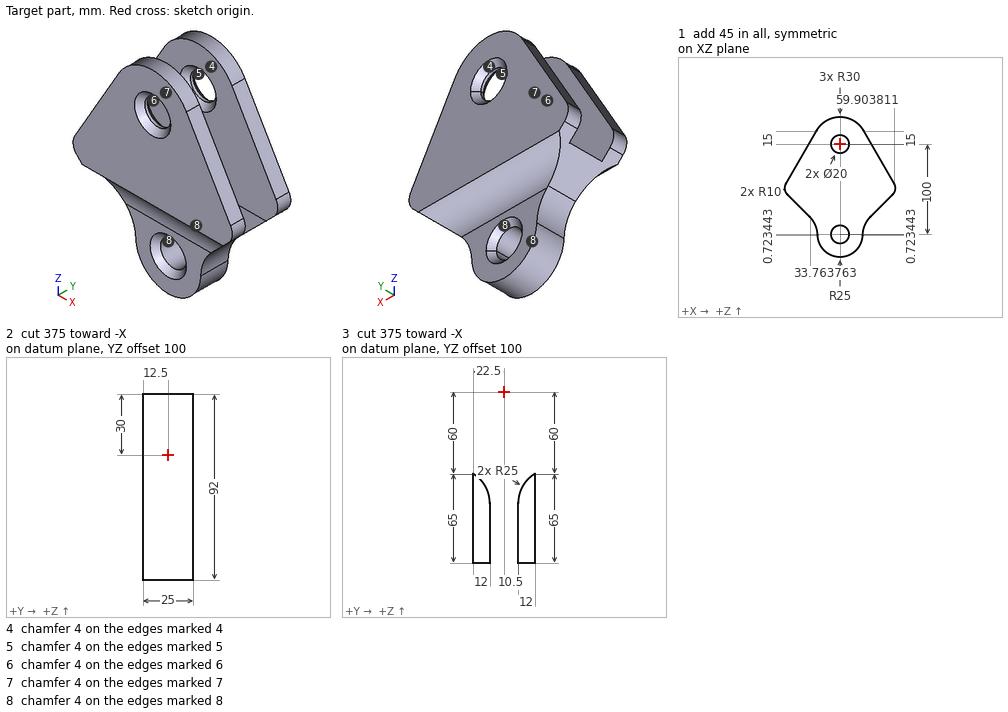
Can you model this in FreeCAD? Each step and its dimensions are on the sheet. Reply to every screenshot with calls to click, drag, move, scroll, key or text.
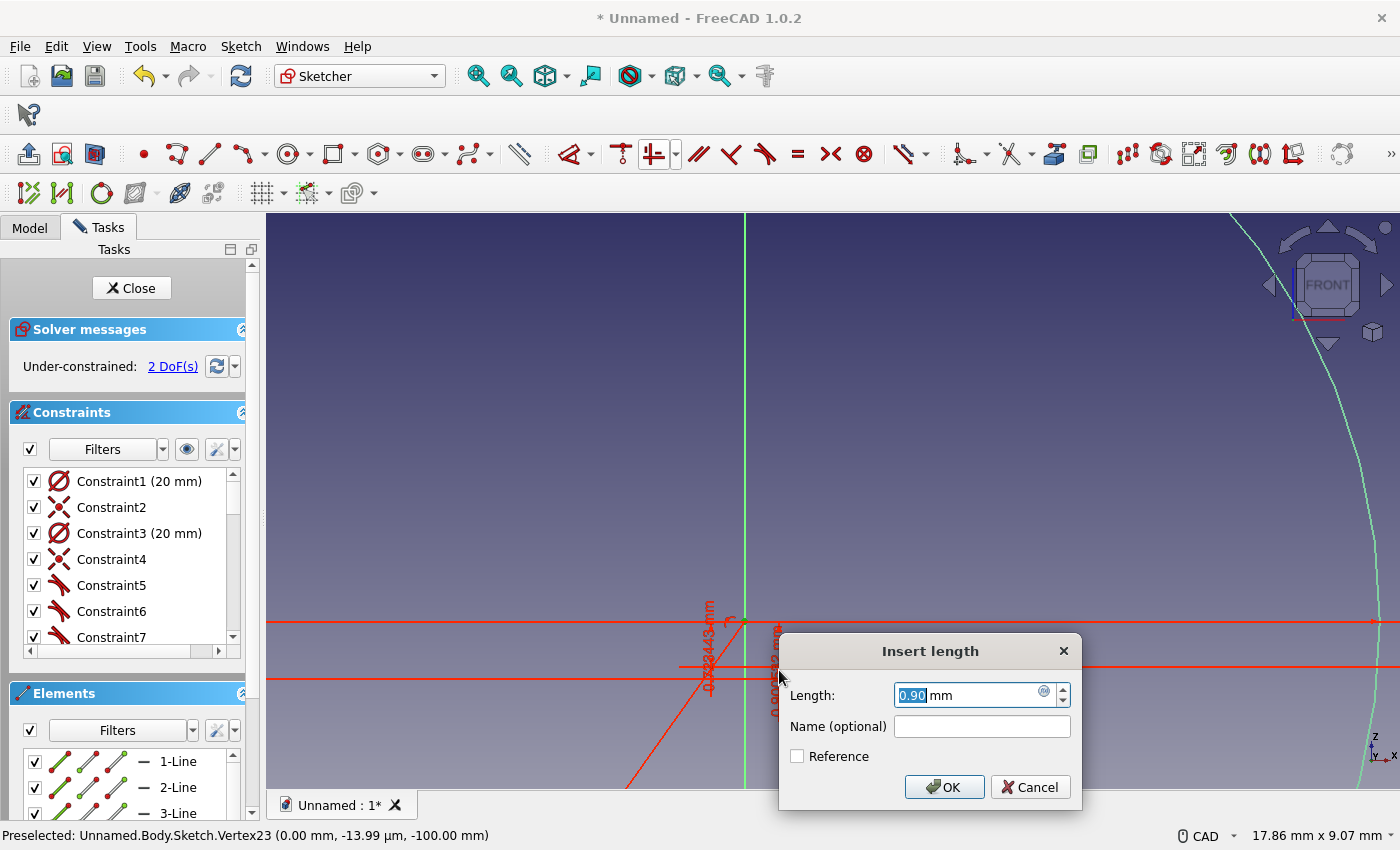
text(0.723443)
key(Return)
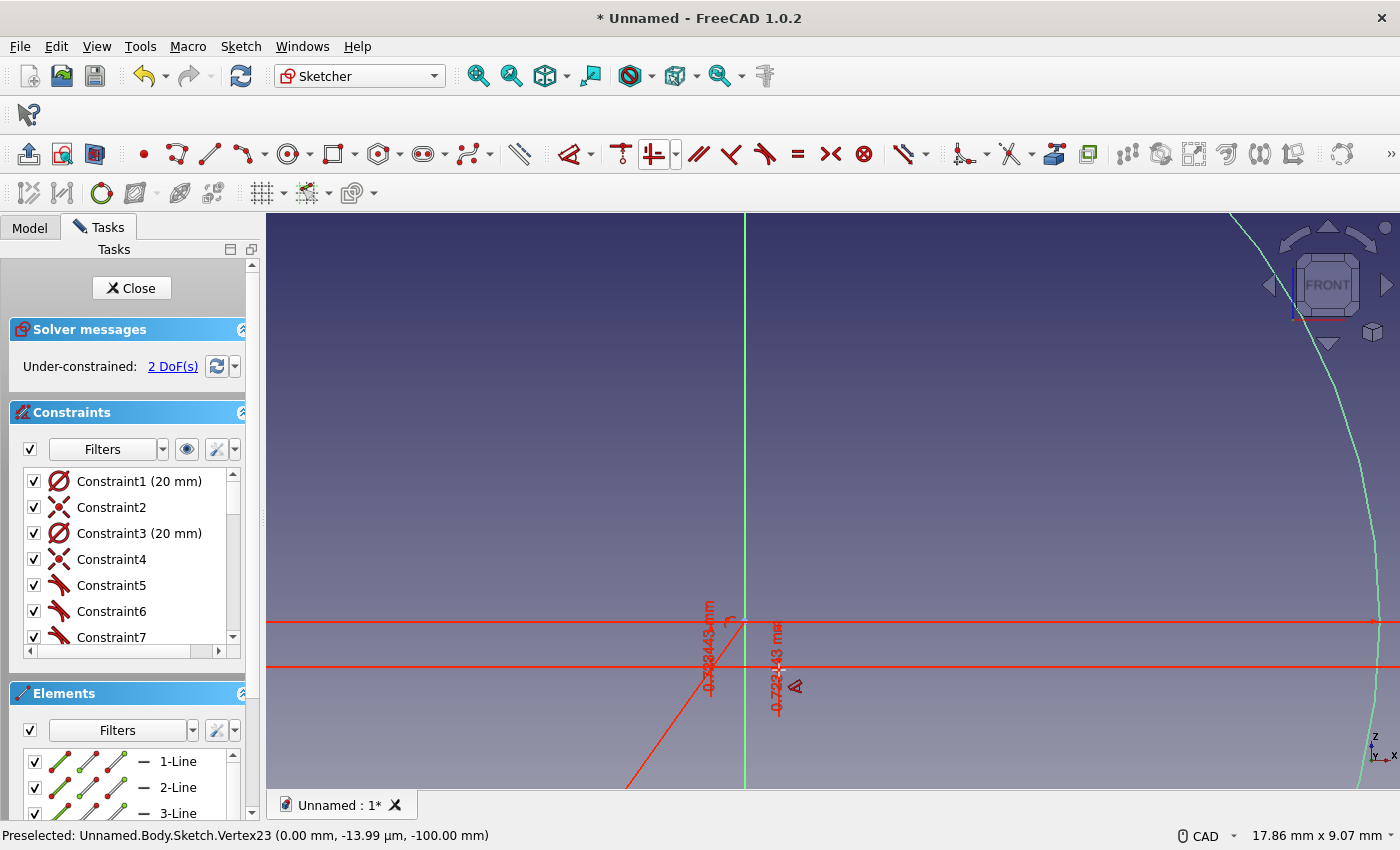
scroll(765, 638, down, 16)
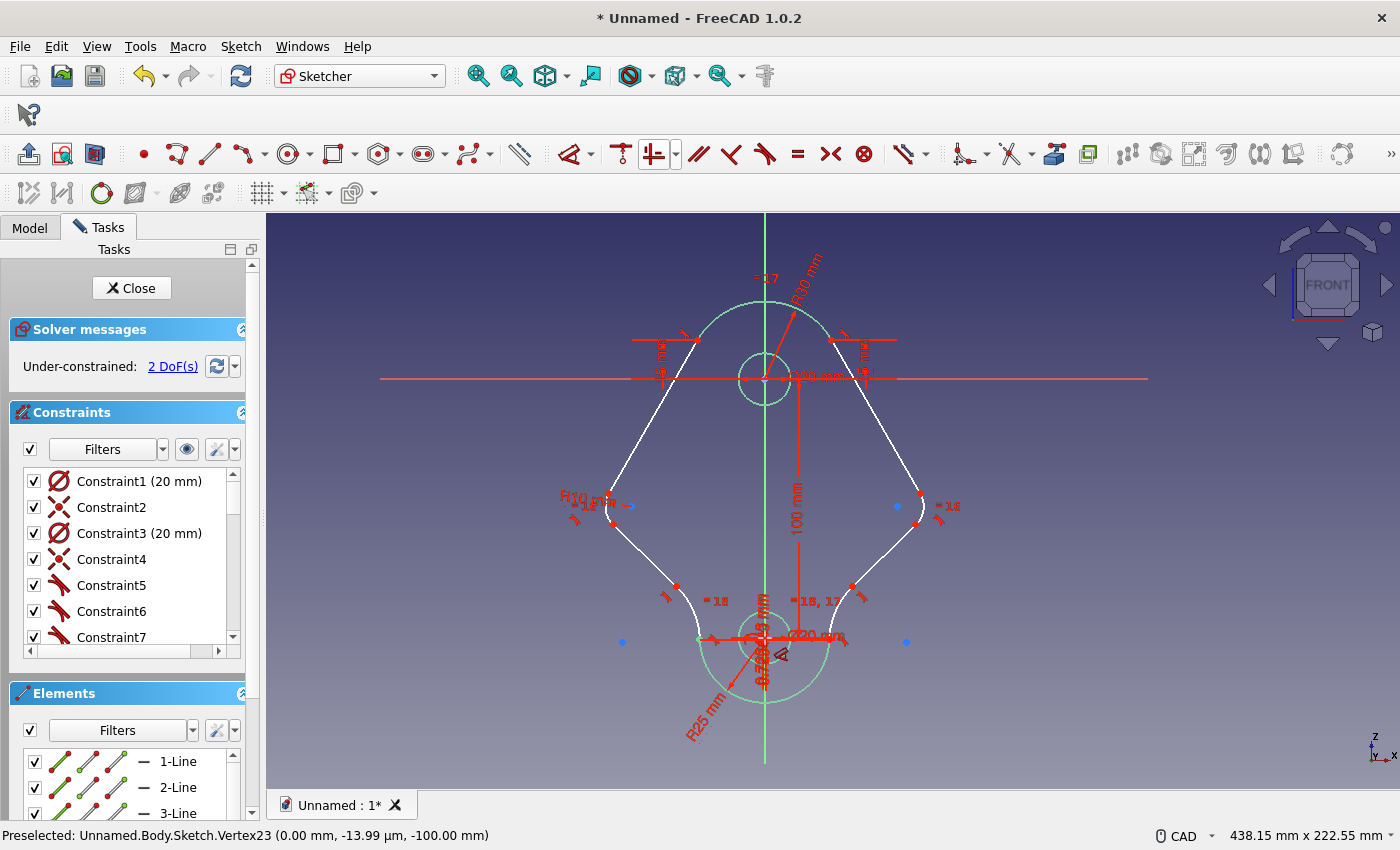
click(677, 587)
click(741, 345)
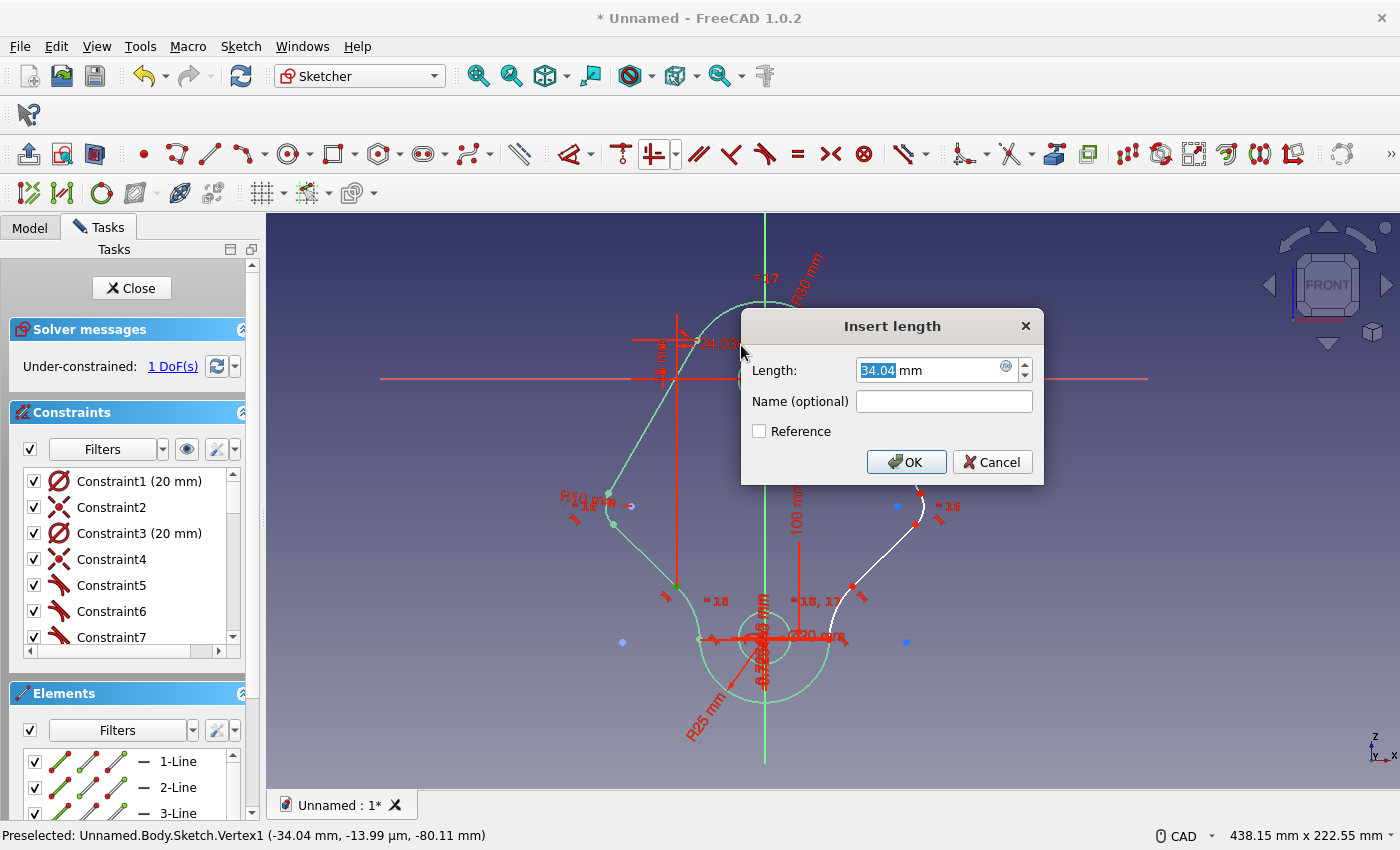
text(33.763763)
key(Return)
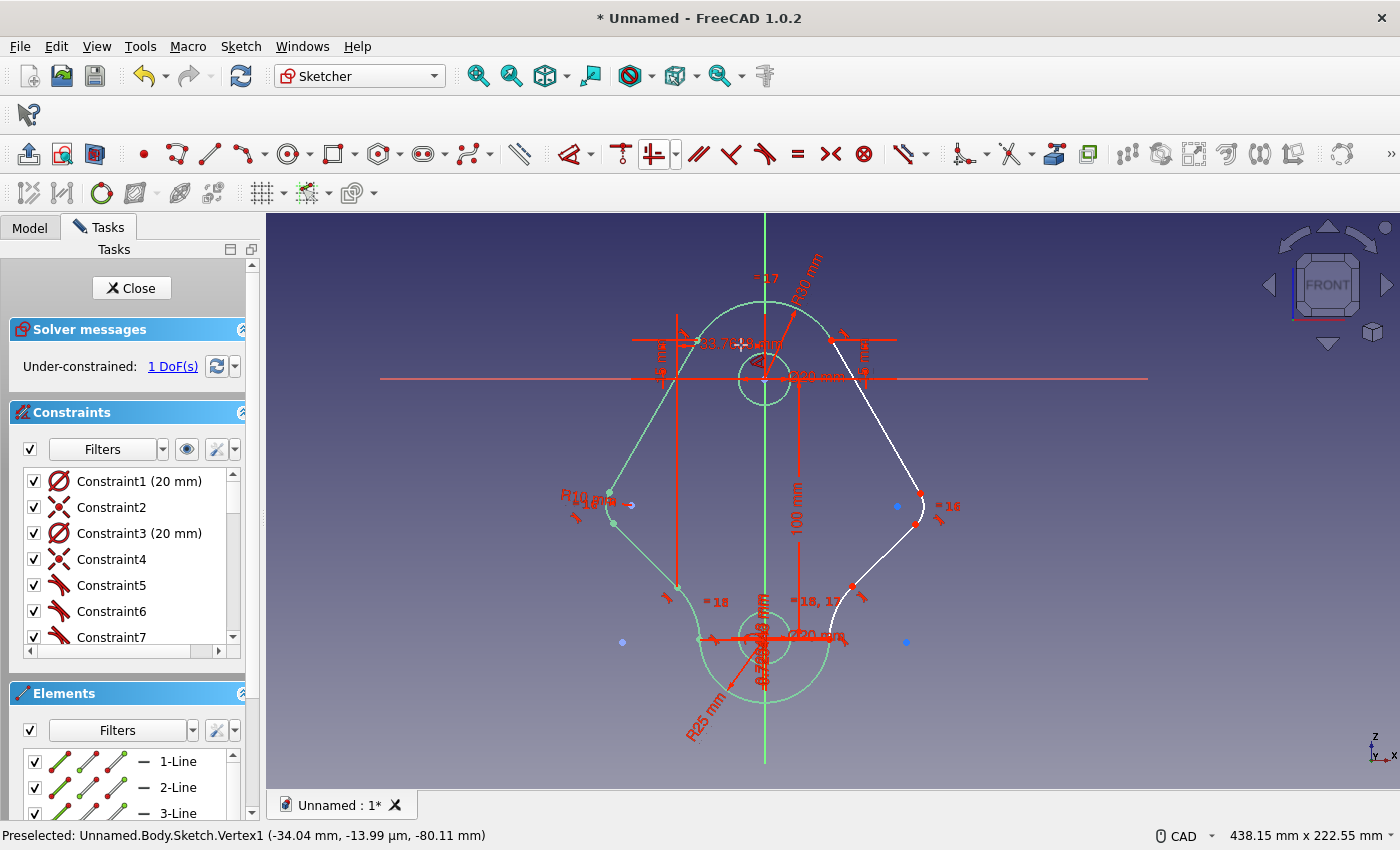
click(920, 493)
click(878, 527)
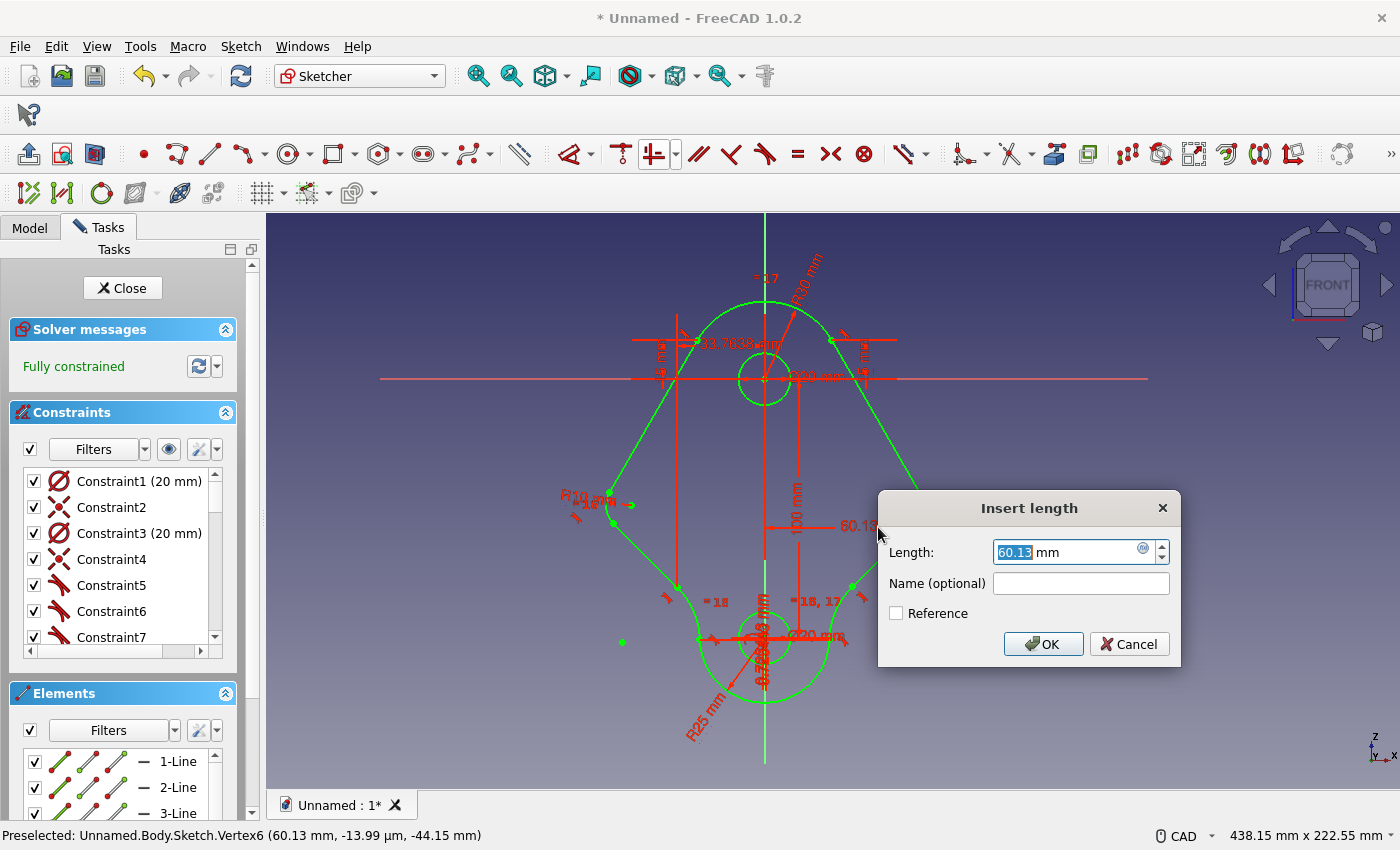
text(59.903811)
key(Return)
key(Escape)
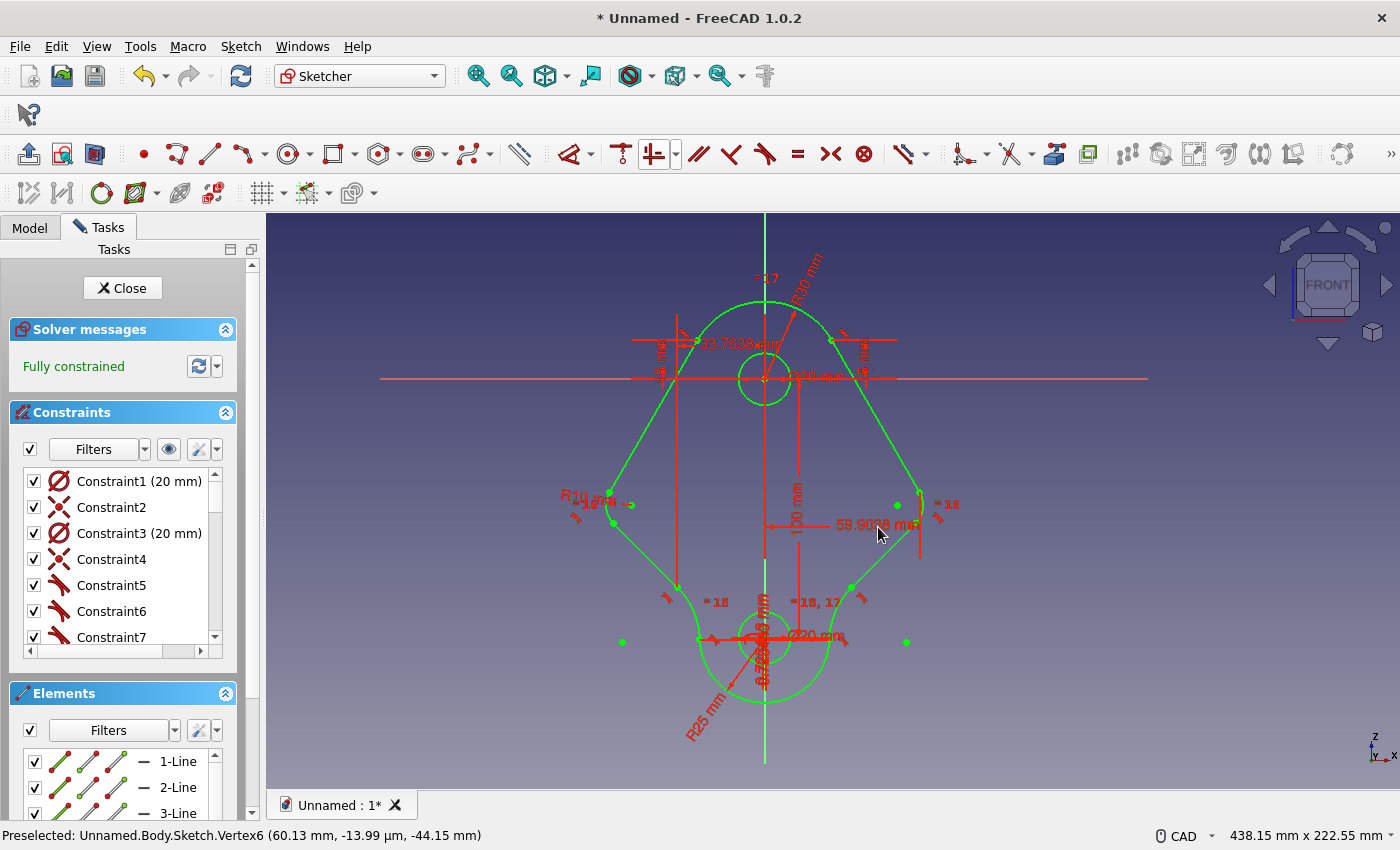
click(123, 288)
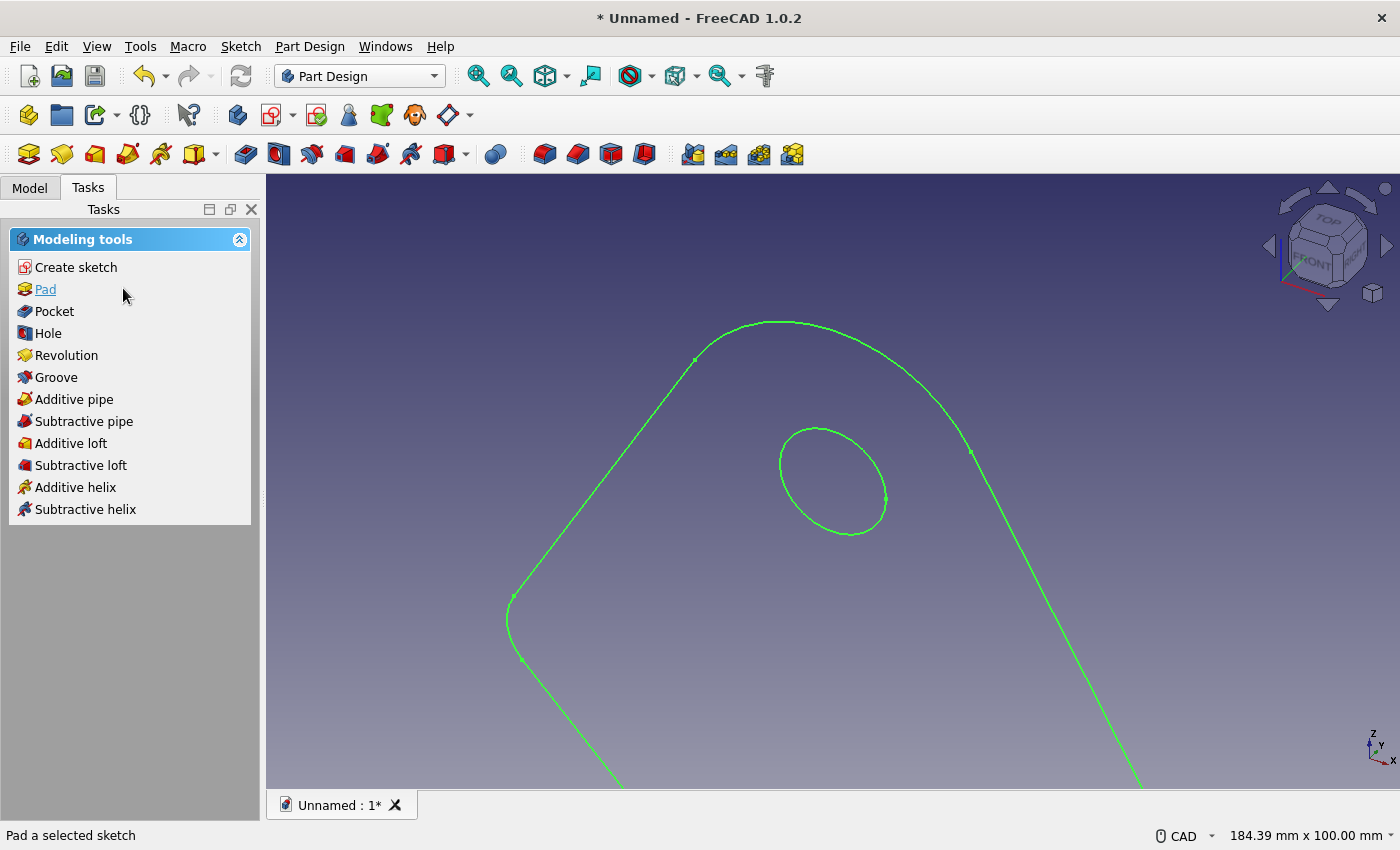
click(29, 154)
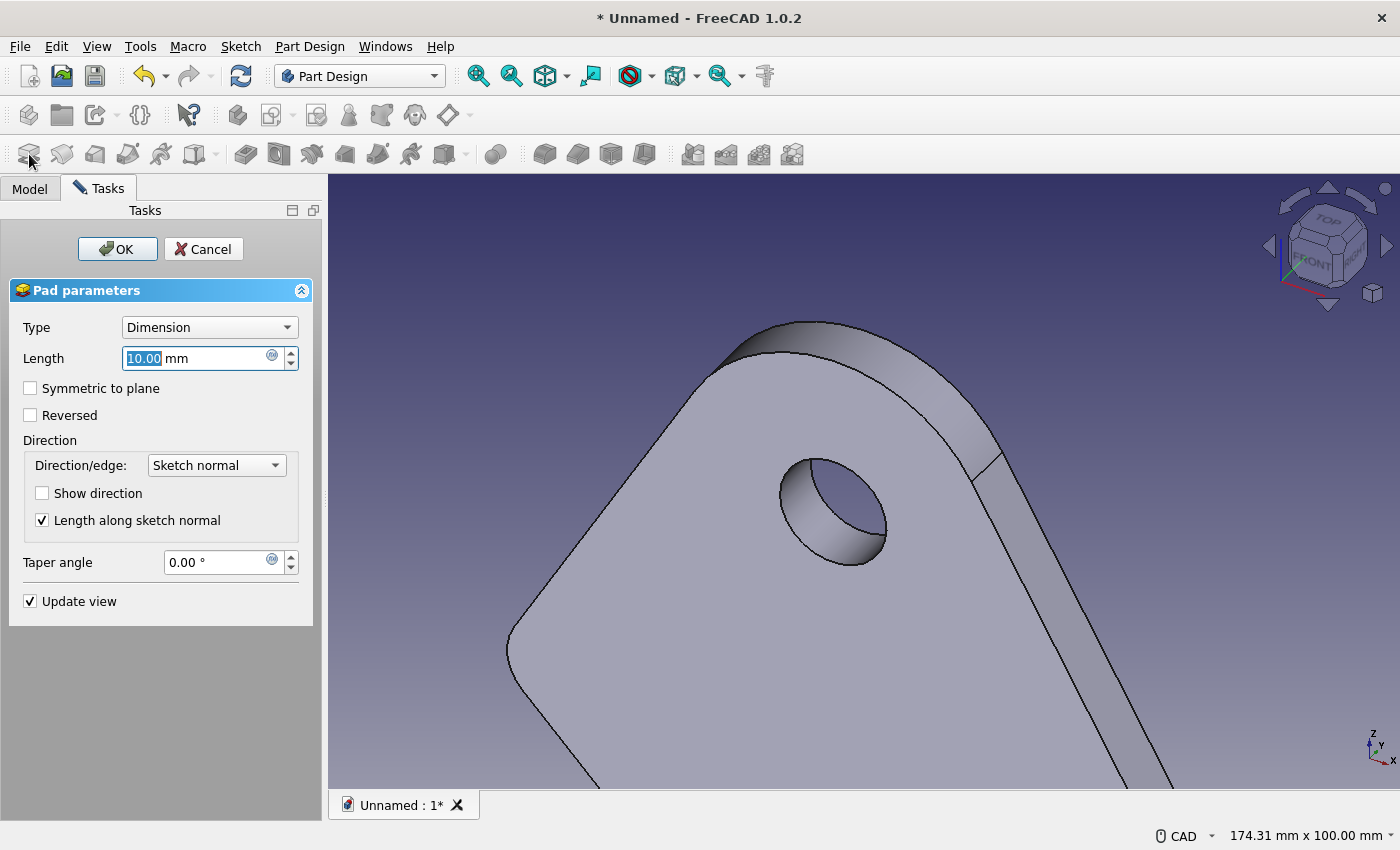
text(45)
key(Tab)